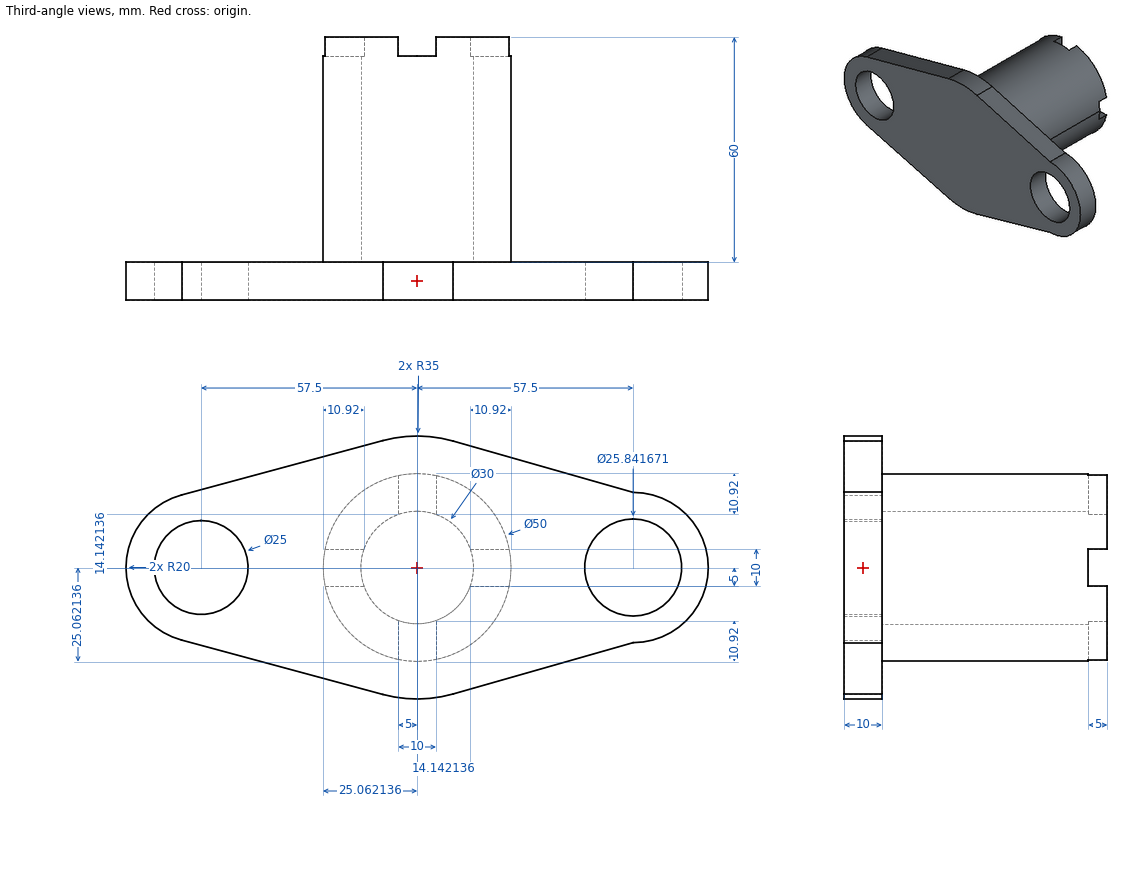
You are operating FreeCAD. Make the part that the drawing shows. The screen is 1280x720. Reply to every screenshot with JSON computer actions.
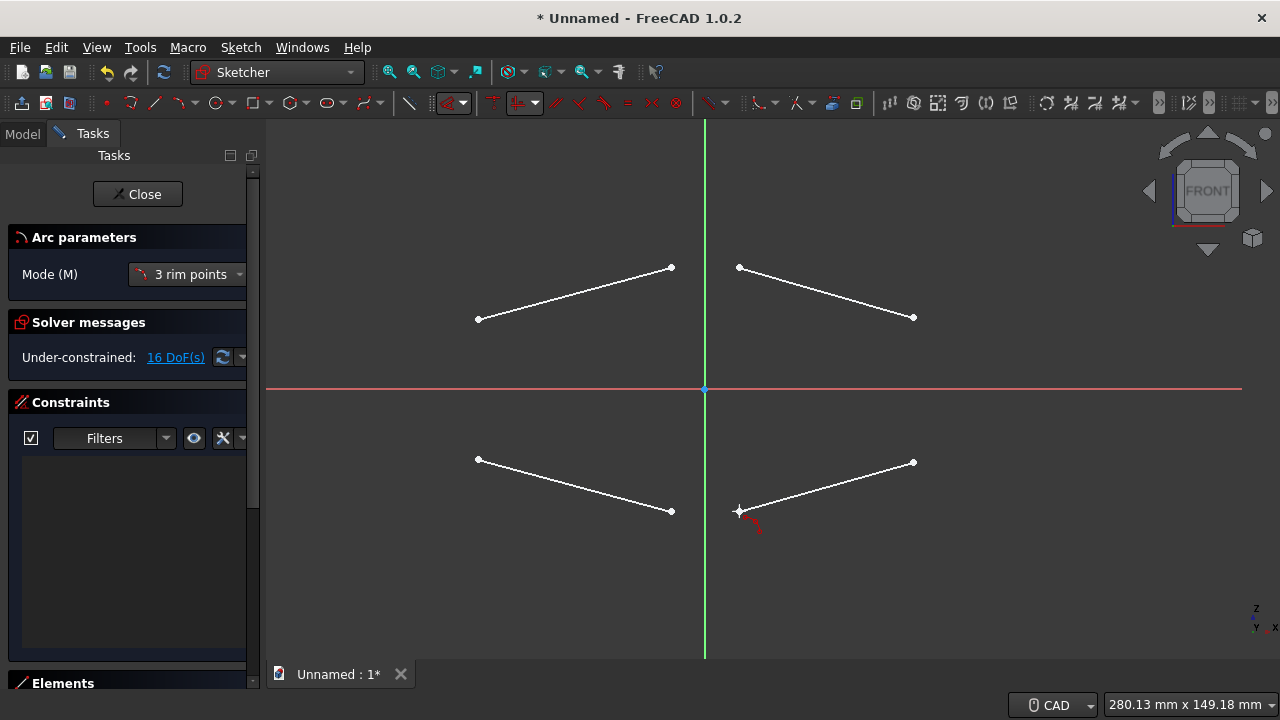
{"action": "left_click", "coordinate": [478, 460]}
{"action": "left_click", "coordinate": [478, 320]}
{"action": "left_click", "coordinate": [426, 370]}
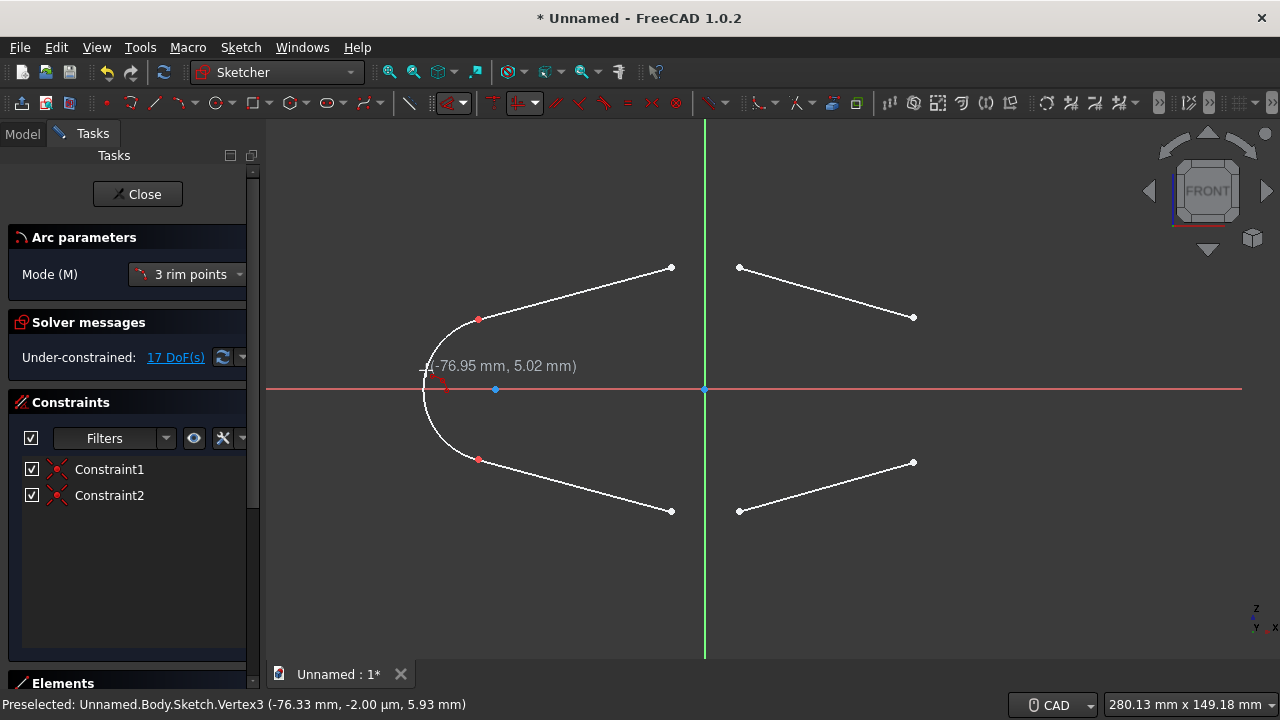
{"action": "left_click", "coordinate": [671, 268]}
{"action": "left_click", "coordinate": [739, 268]}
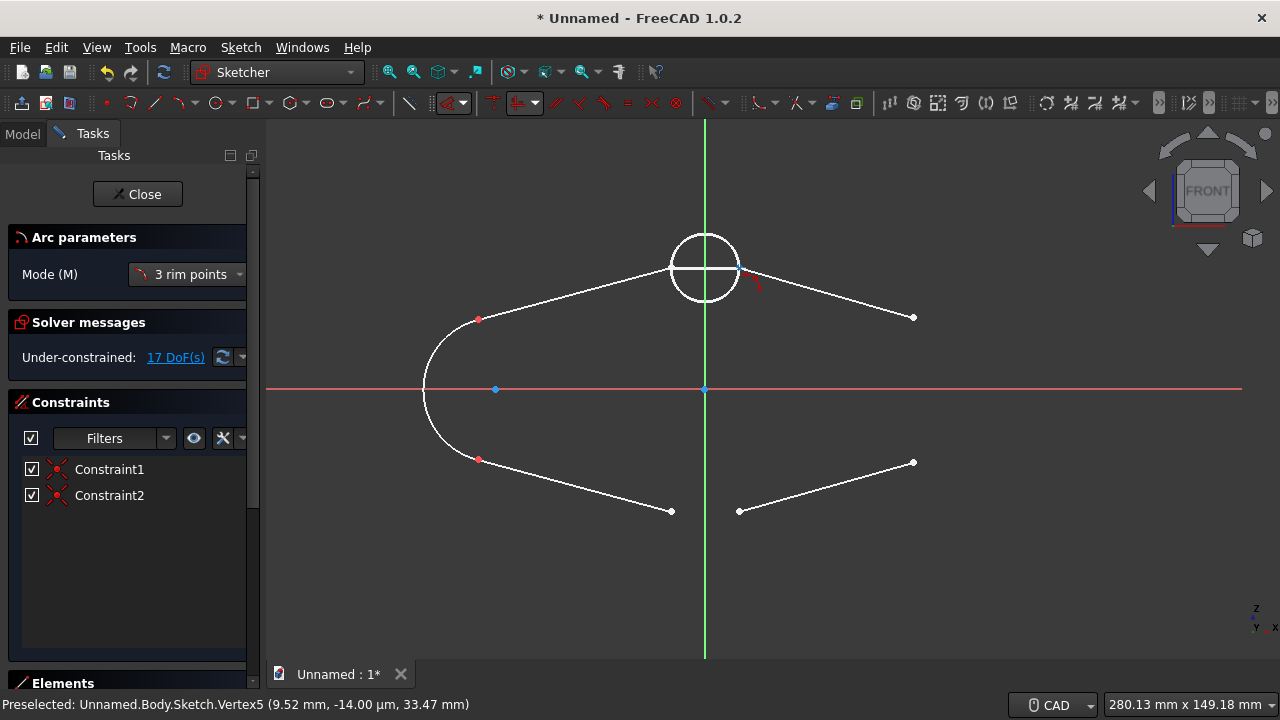
{"action": "scroll", "coordinate": [699, 263], "scroll_direction": "up", "scroll_amount": 7}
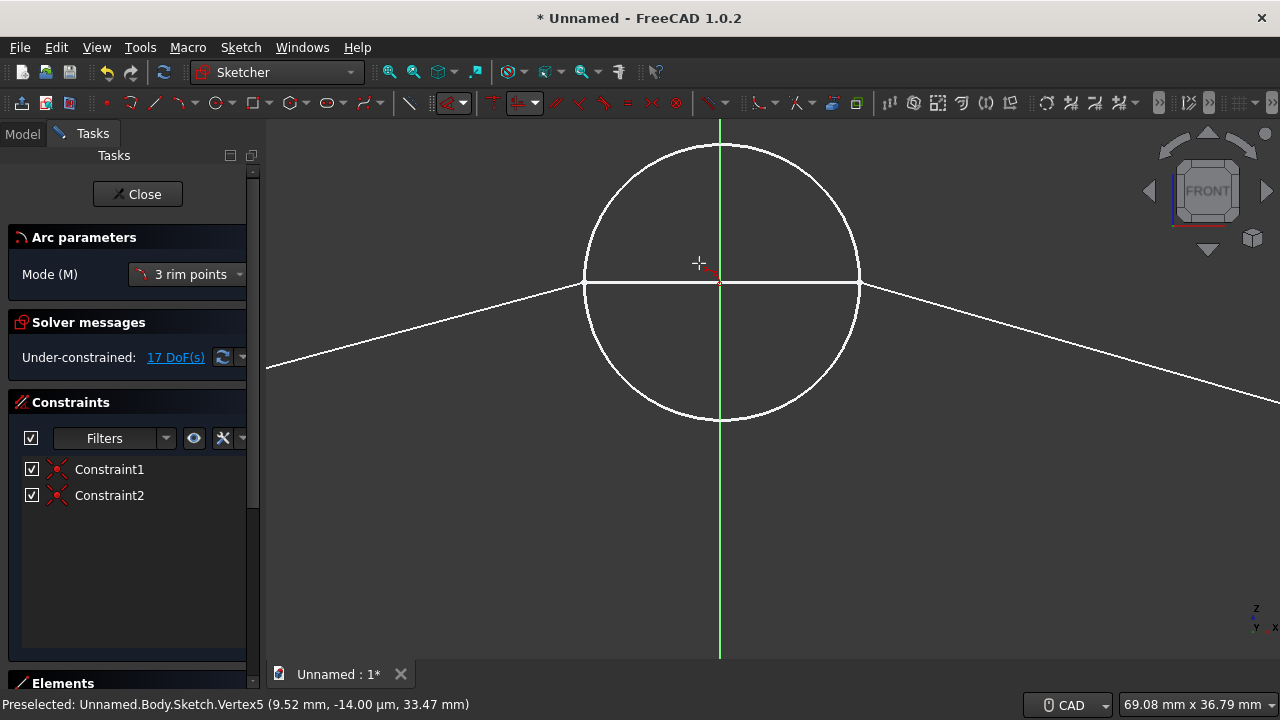
{"action": "left_click", "coordinate": [696, 261]}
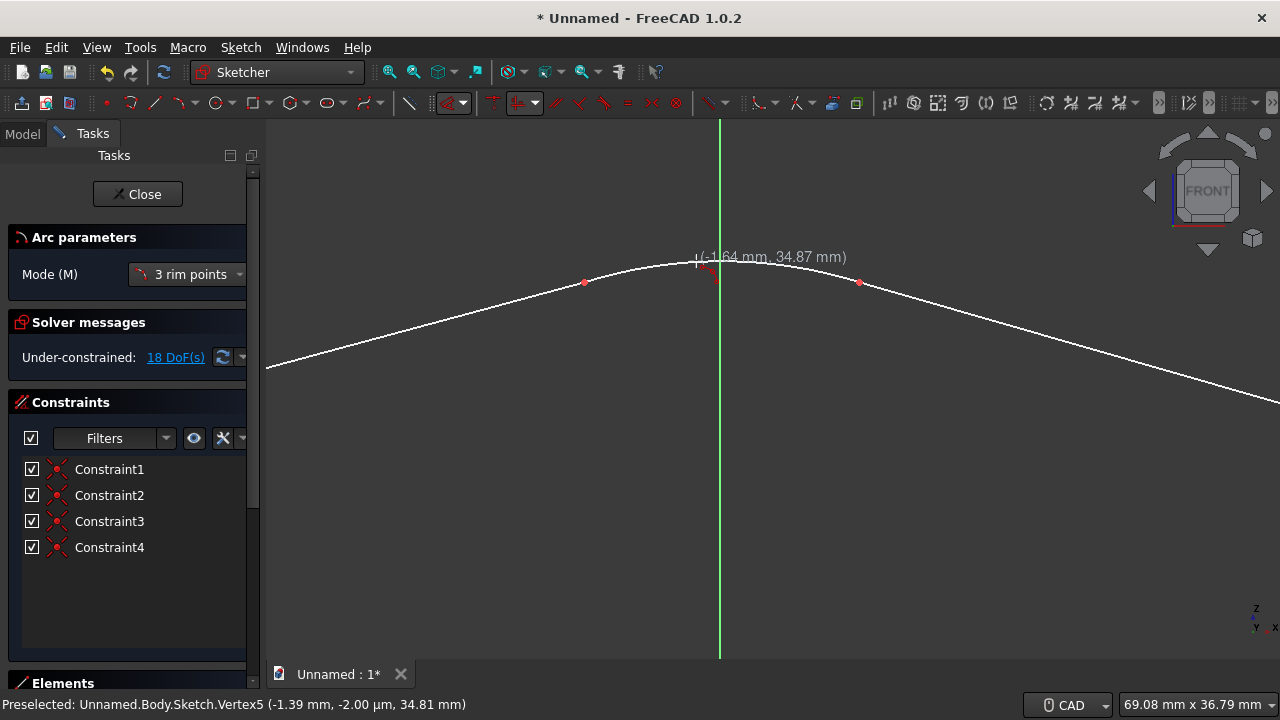
{"action": "scroll", "coordinate": [699, 263], "scroll_direction": "down", "scroll_amount": 7}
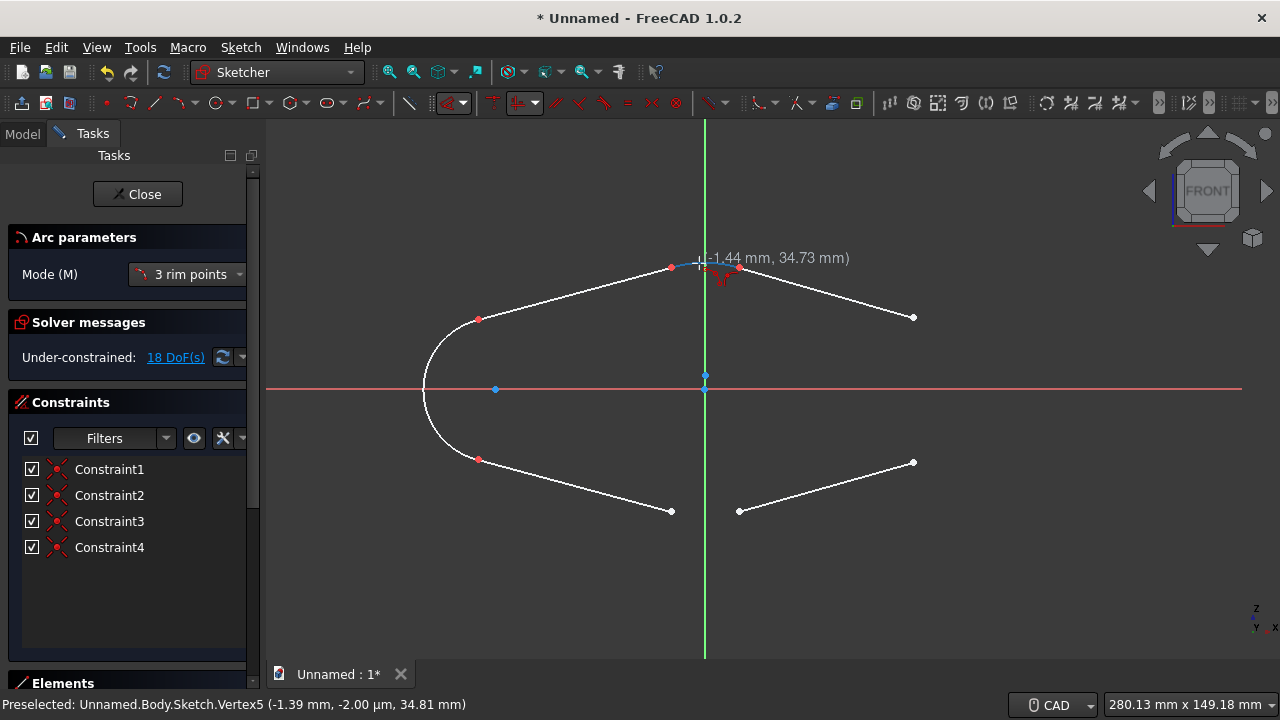
{"action": "left_click", "coordinate": [913, 318]}
{"action": "left_click", "coordinate": [913, 463]}
{"action": "left_click", "coordinate": [982, 412]}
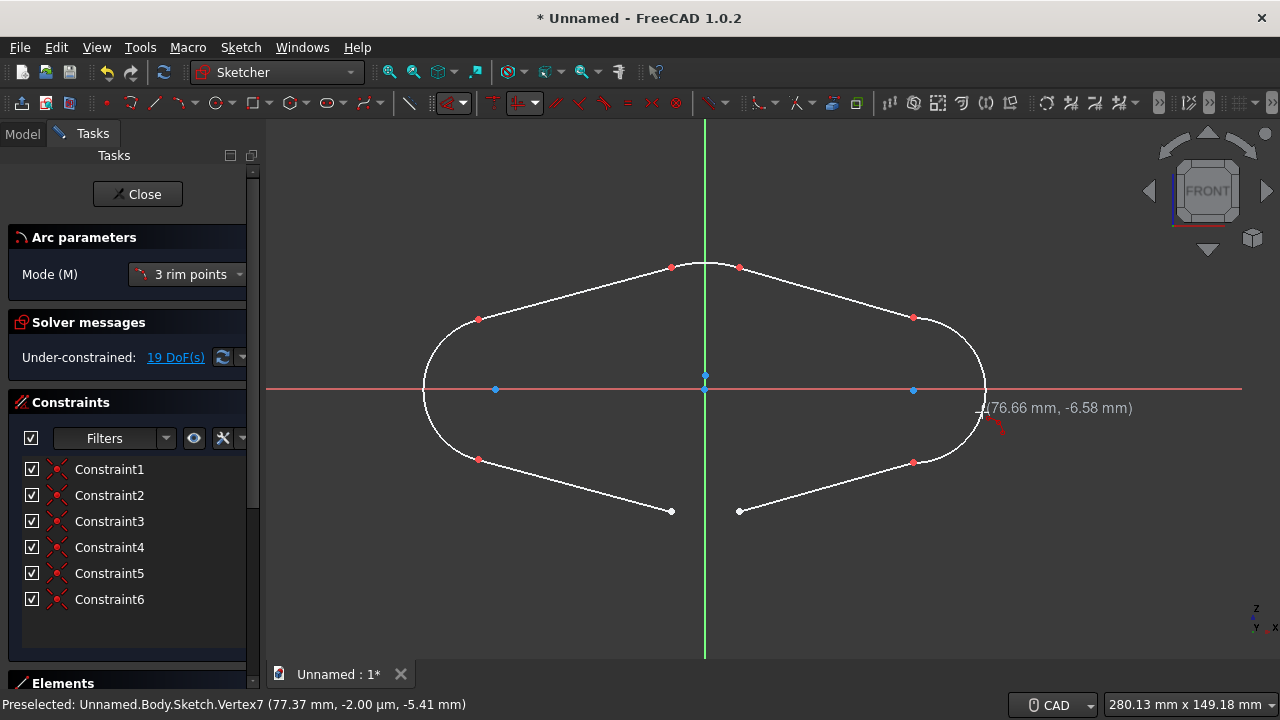
{"action": "left_click", "coordinate": [739, 512]}
{"action": "left_click", "coordinate": [671, 512]}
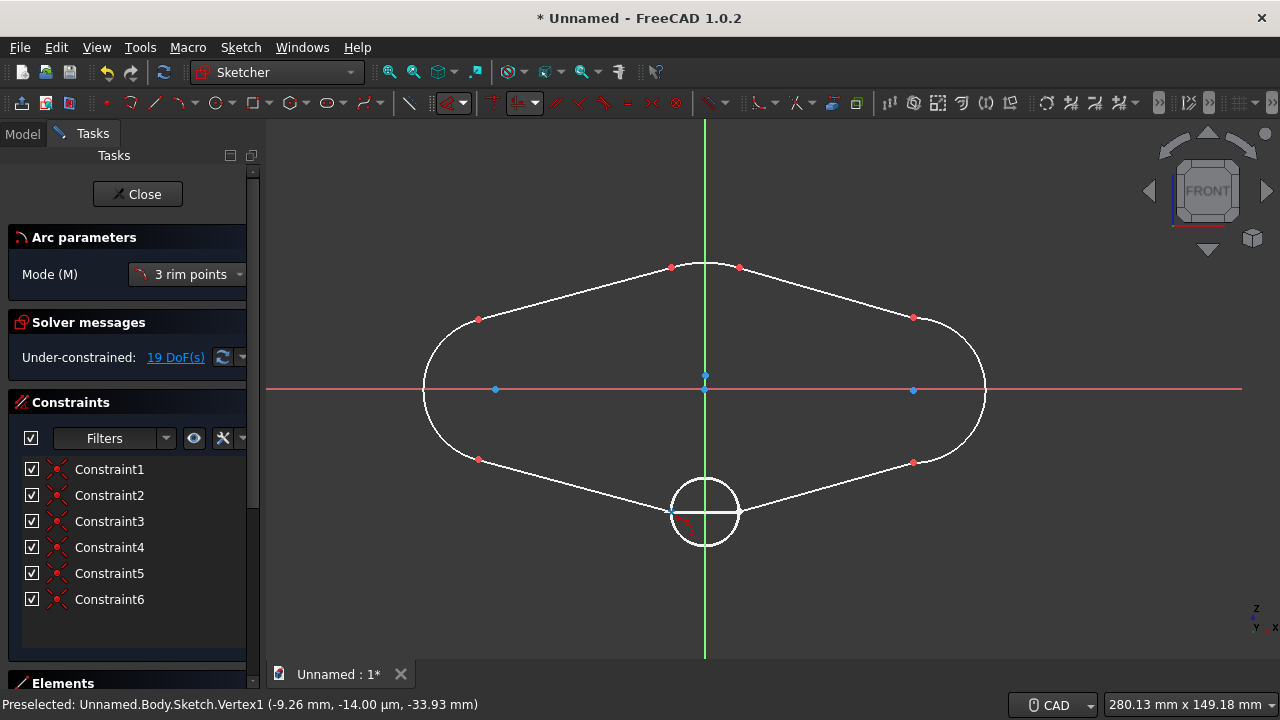
{"action": "scroll", "coordinate": [699, 516], "scroll_direction": "up", "scroll_amount": 7}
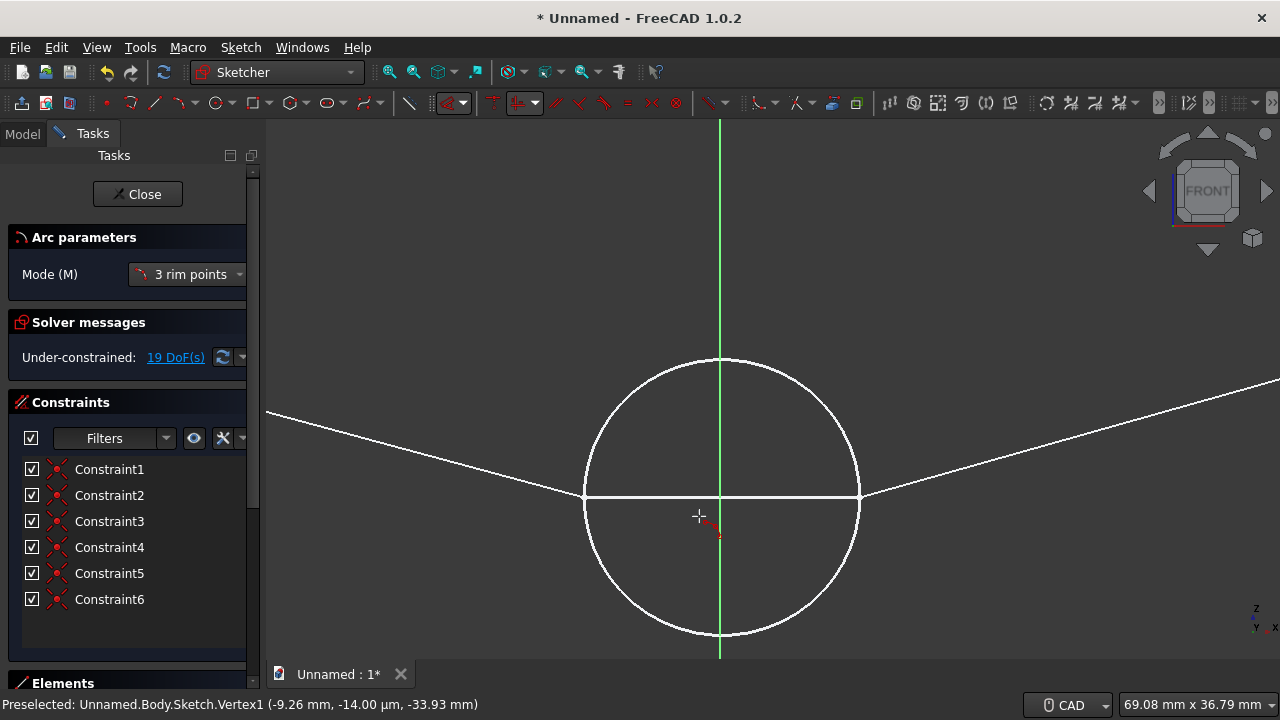
{"action": "left_click", "coordinate": [696, 513]}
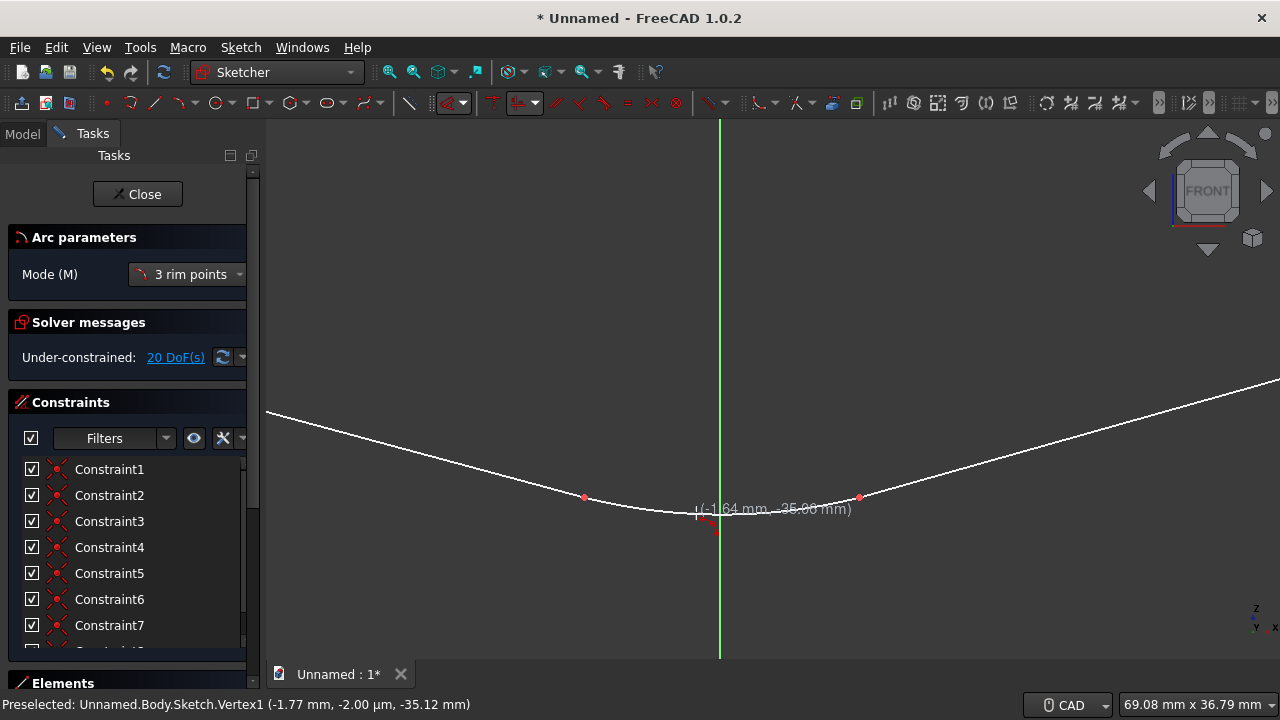
{"action": "key", "text": "g c"}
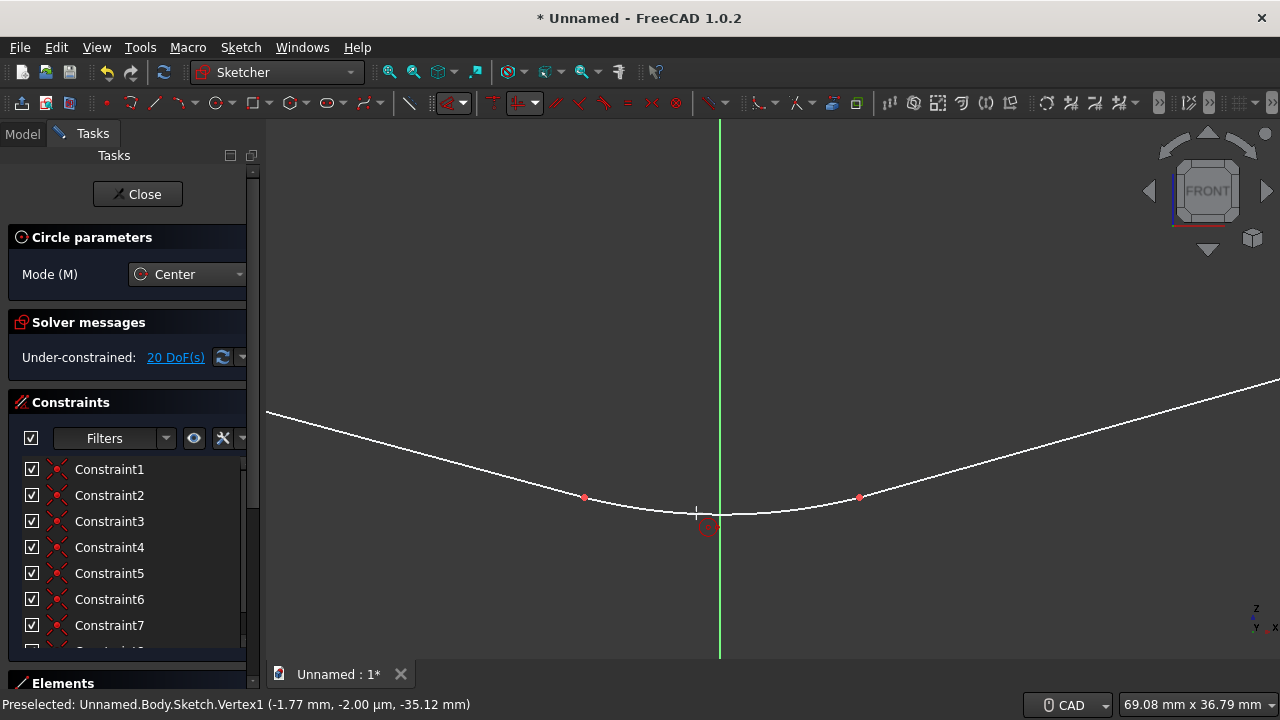
{"action": "scroll", "coordinate": [699, 517], "scroll_direction": "down", "scroll_amount": 7}